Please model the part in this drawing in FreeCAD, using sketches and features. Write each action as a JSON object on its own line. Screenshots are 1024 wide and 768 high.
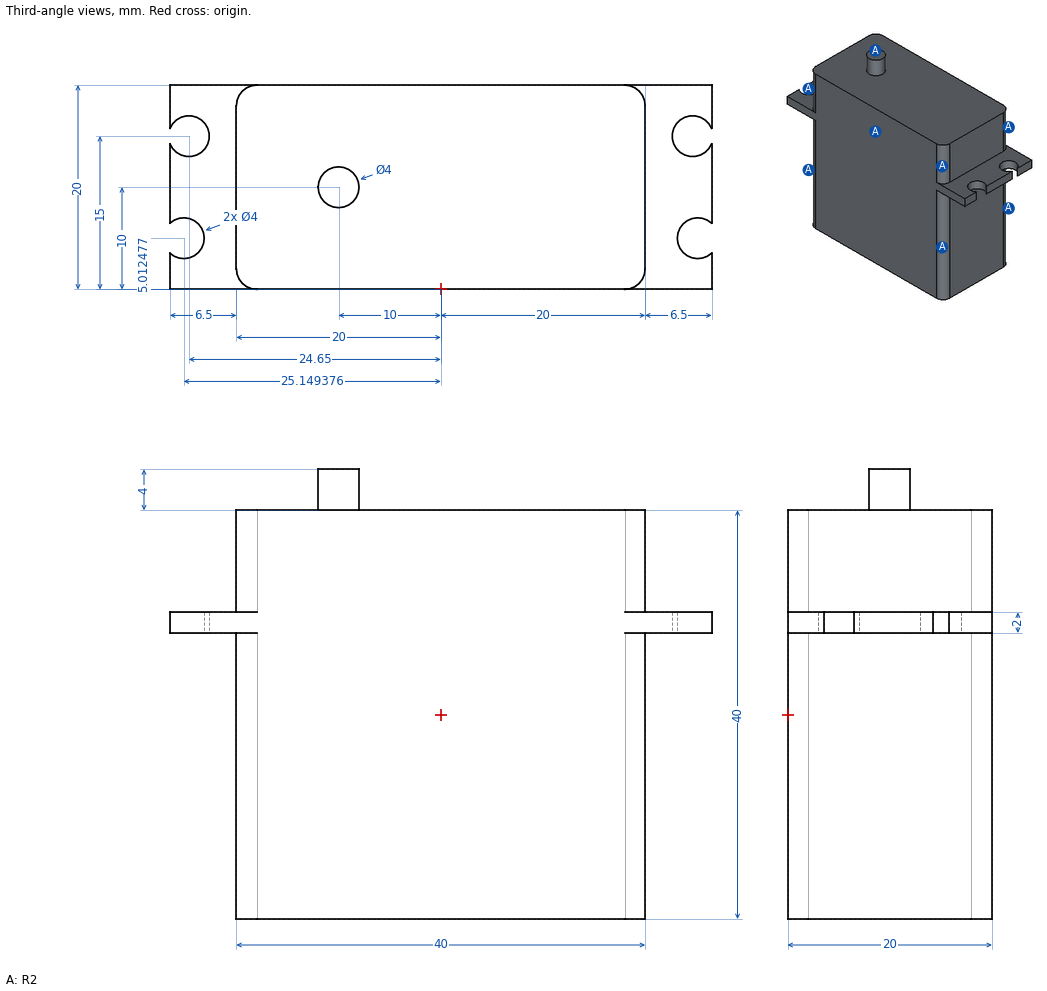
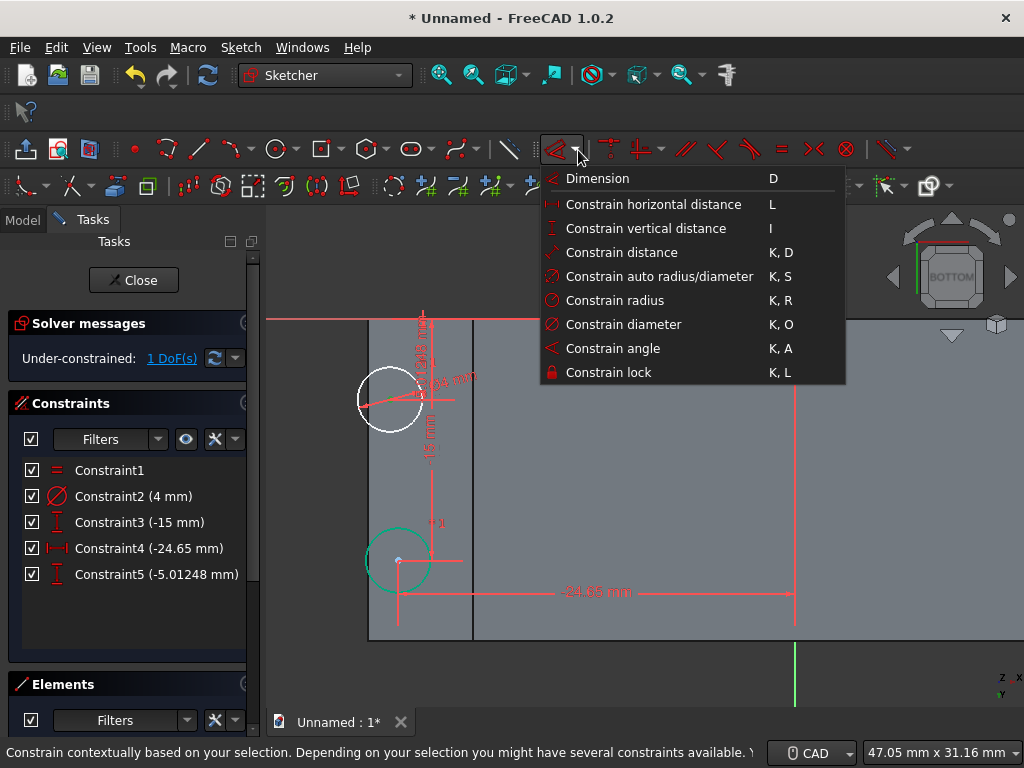
{"action": "left_click", "coordinate": [693, 204]}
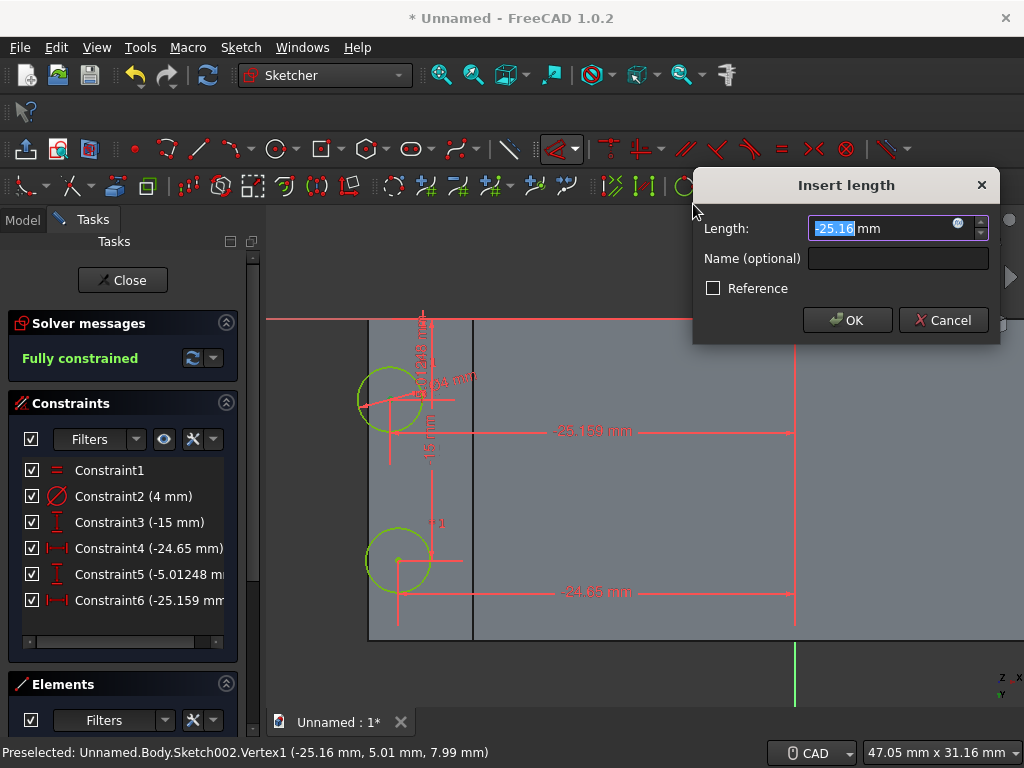
{"action": "type", "text": "-25.149376"}
{"action": "key", "text": "Return"}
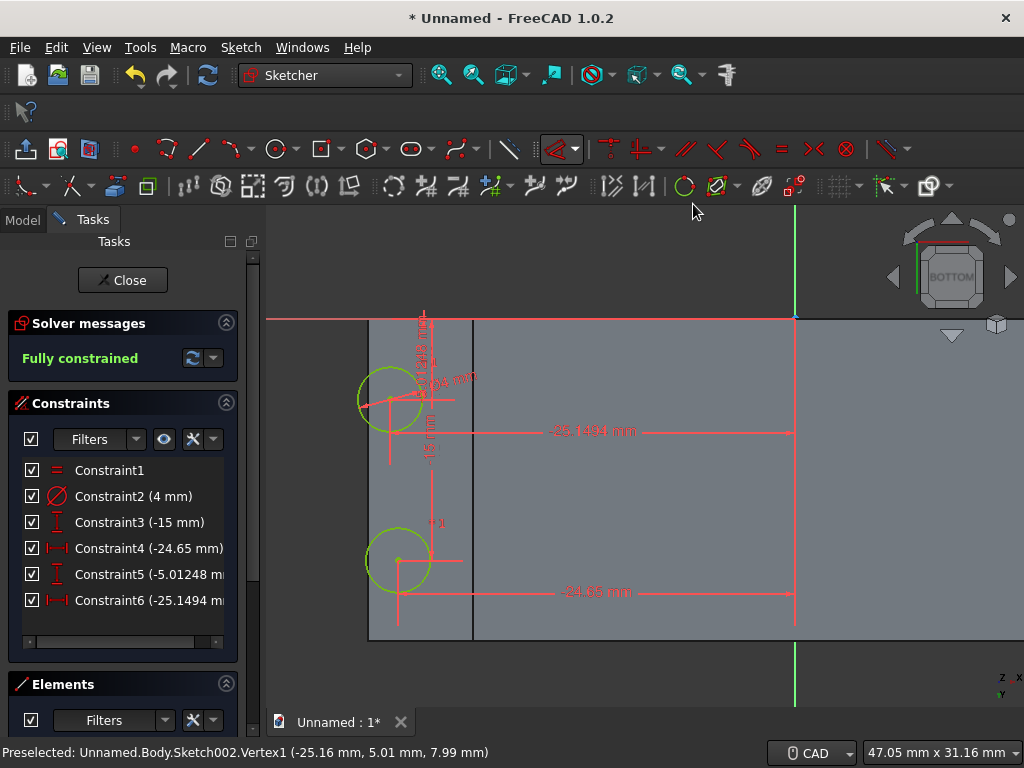
{"action": "left_click", "coordinate": [123, 280]}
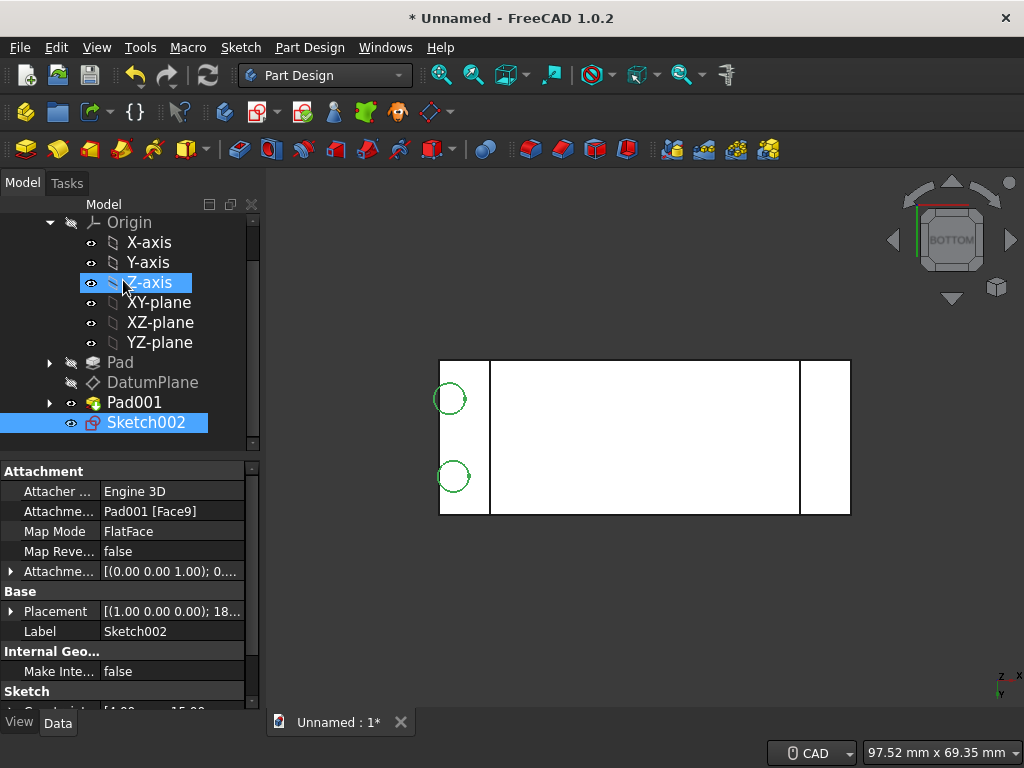
{"action": "left_click", "coordinate": [240, 150]}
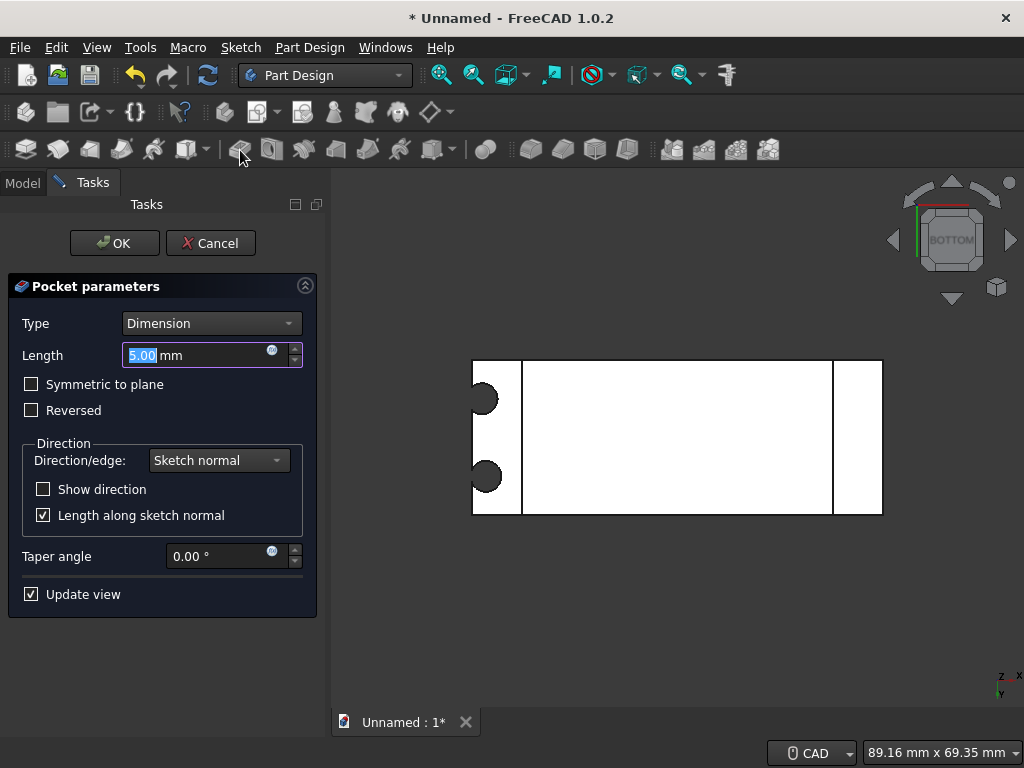
{"action": "type", "text": "2"}
{"action": "key", "text": "Tab"}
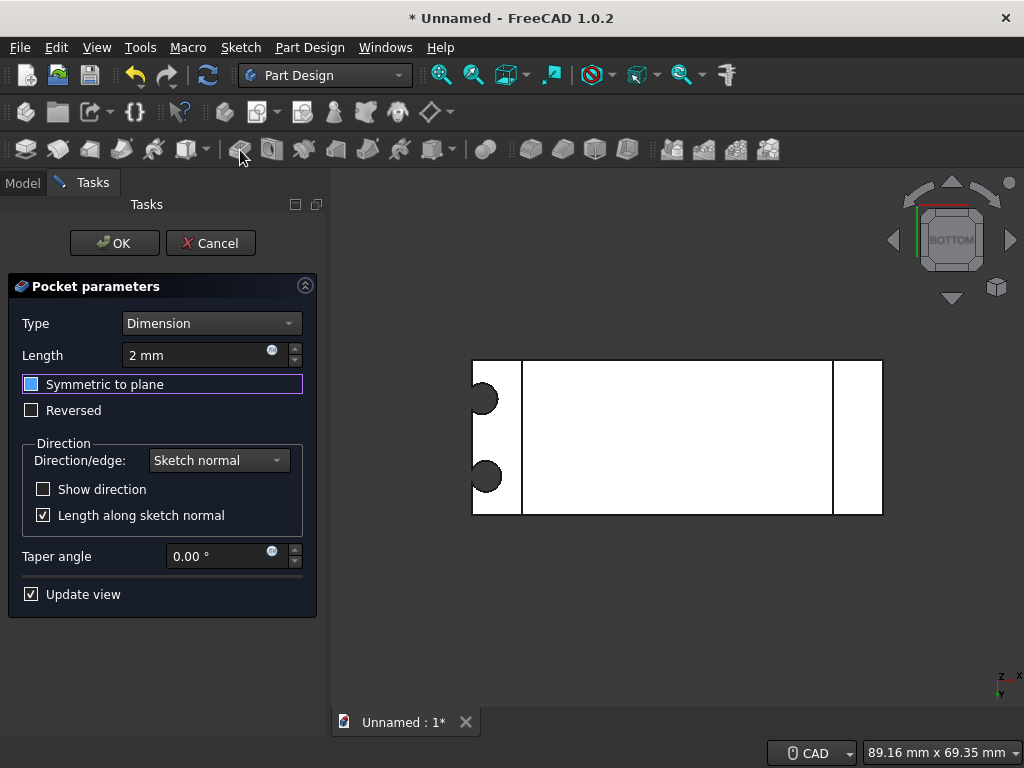
{"action": "left_click", "coordinate": [115, 243]}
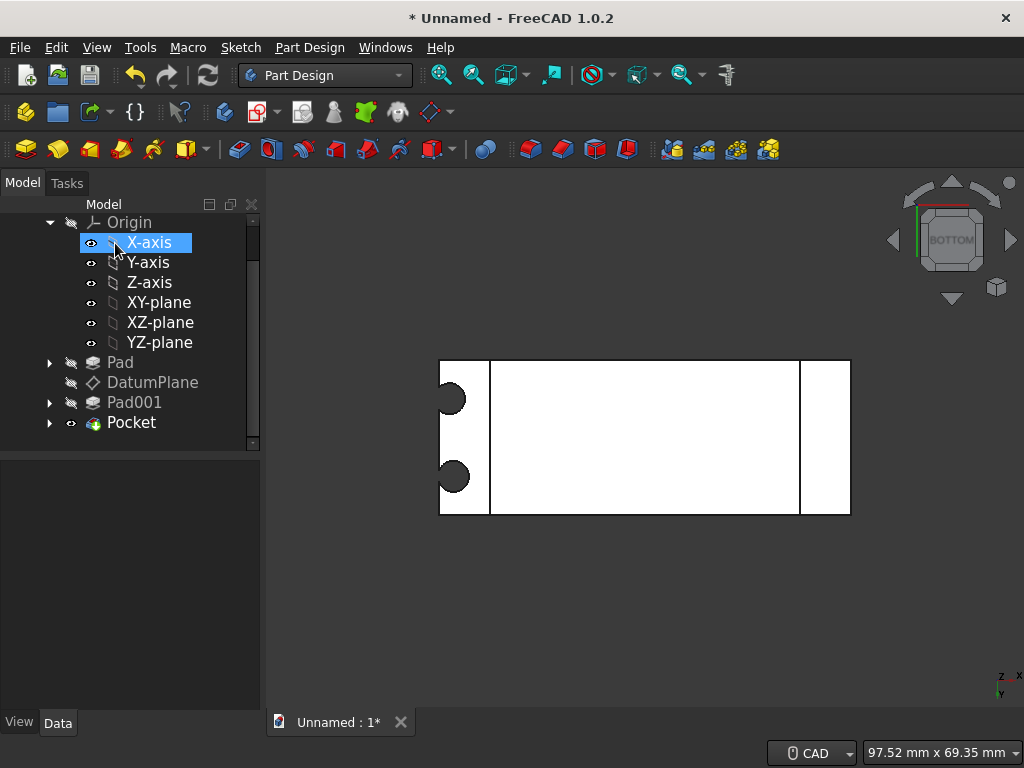
{"action": "left_click", "coordinate": [116, 423]}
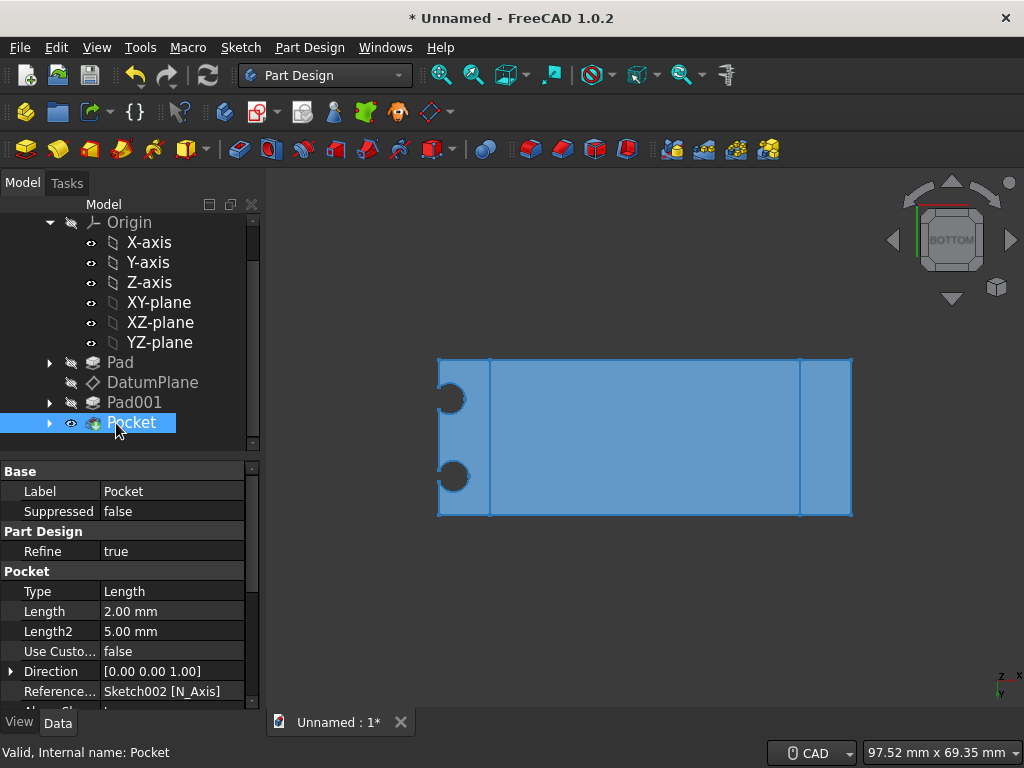
{"action": "left_click", "coordinate": [672, 150]}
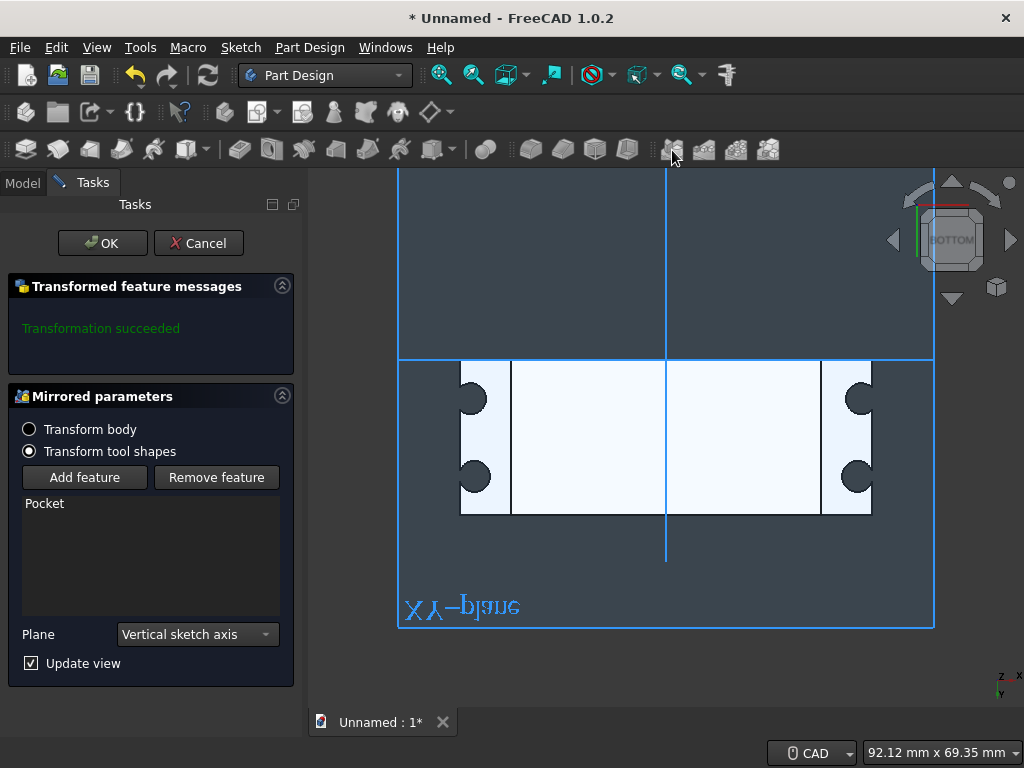
{"action": "left_click", "coordinate": [198, 634]}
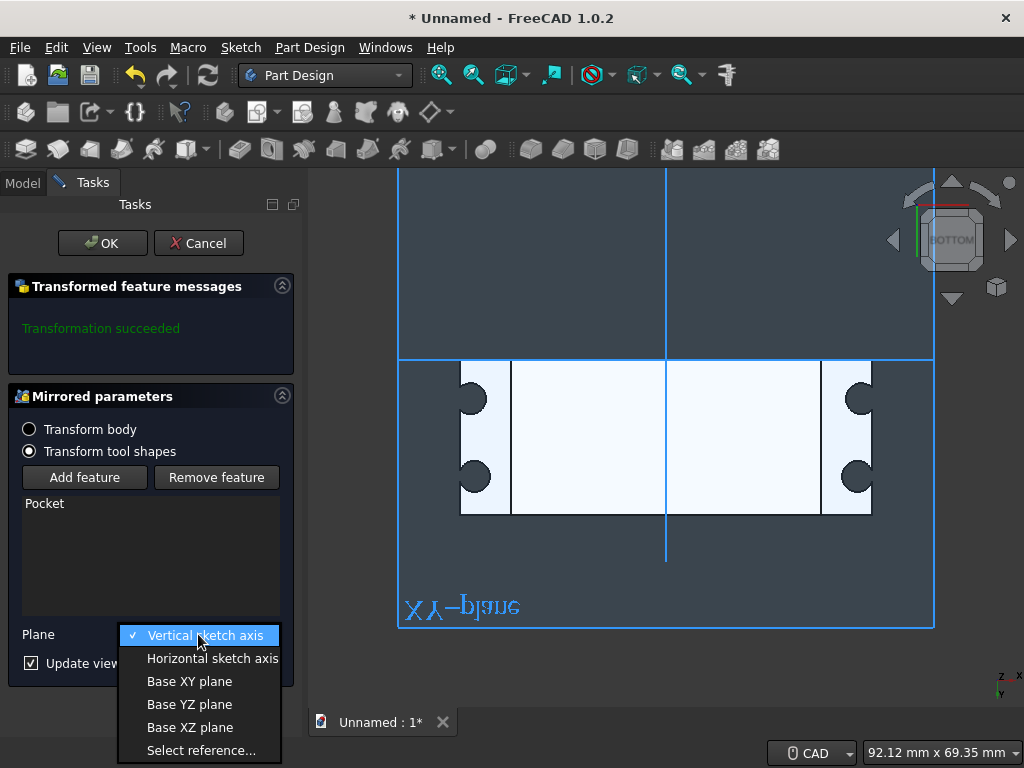
{"action": "left_click", "coordinate": [198, 704]}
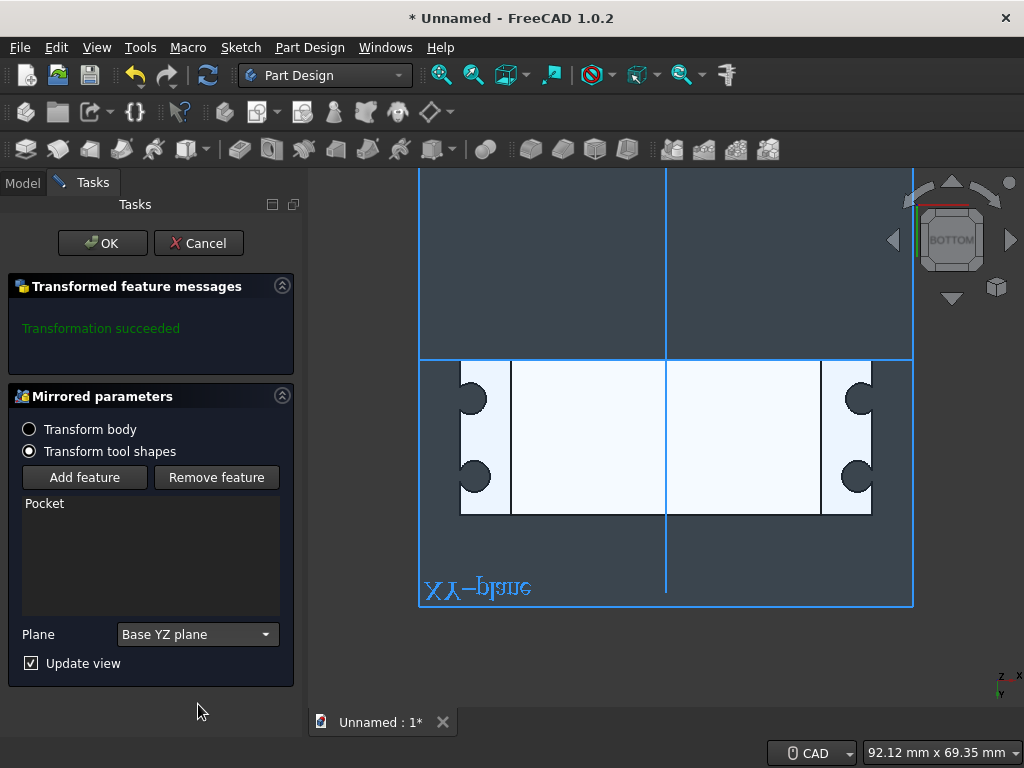
{"action": "left_click", "coordinate": [103, 243]}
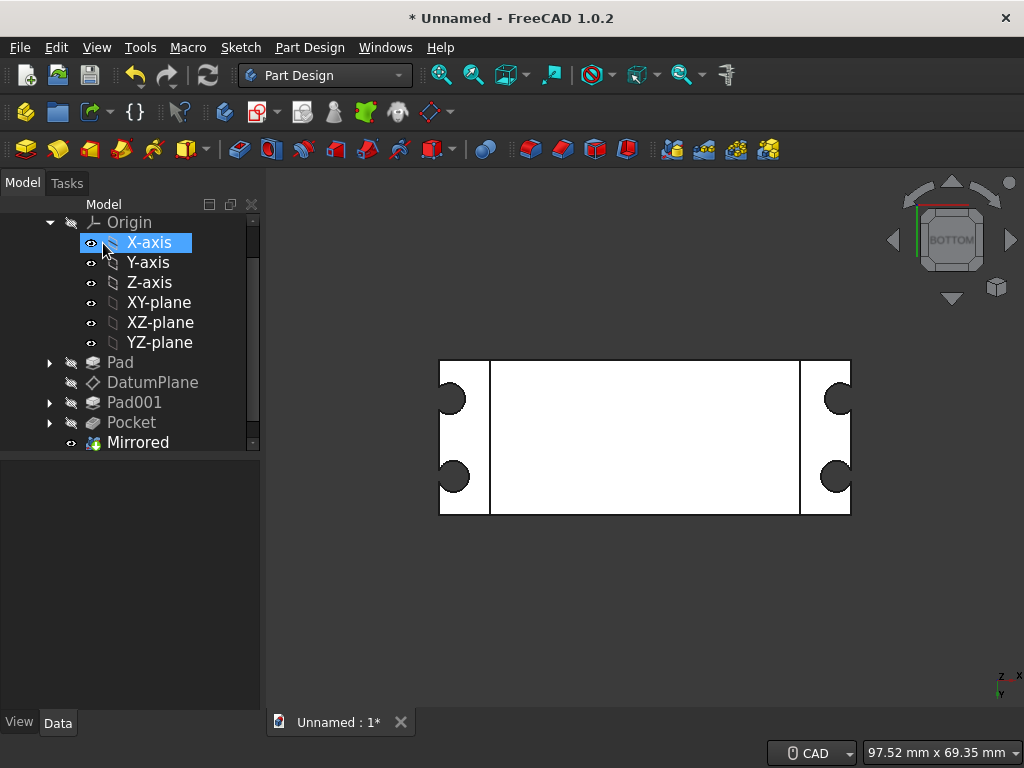
{"action": "key", "text": "0"}